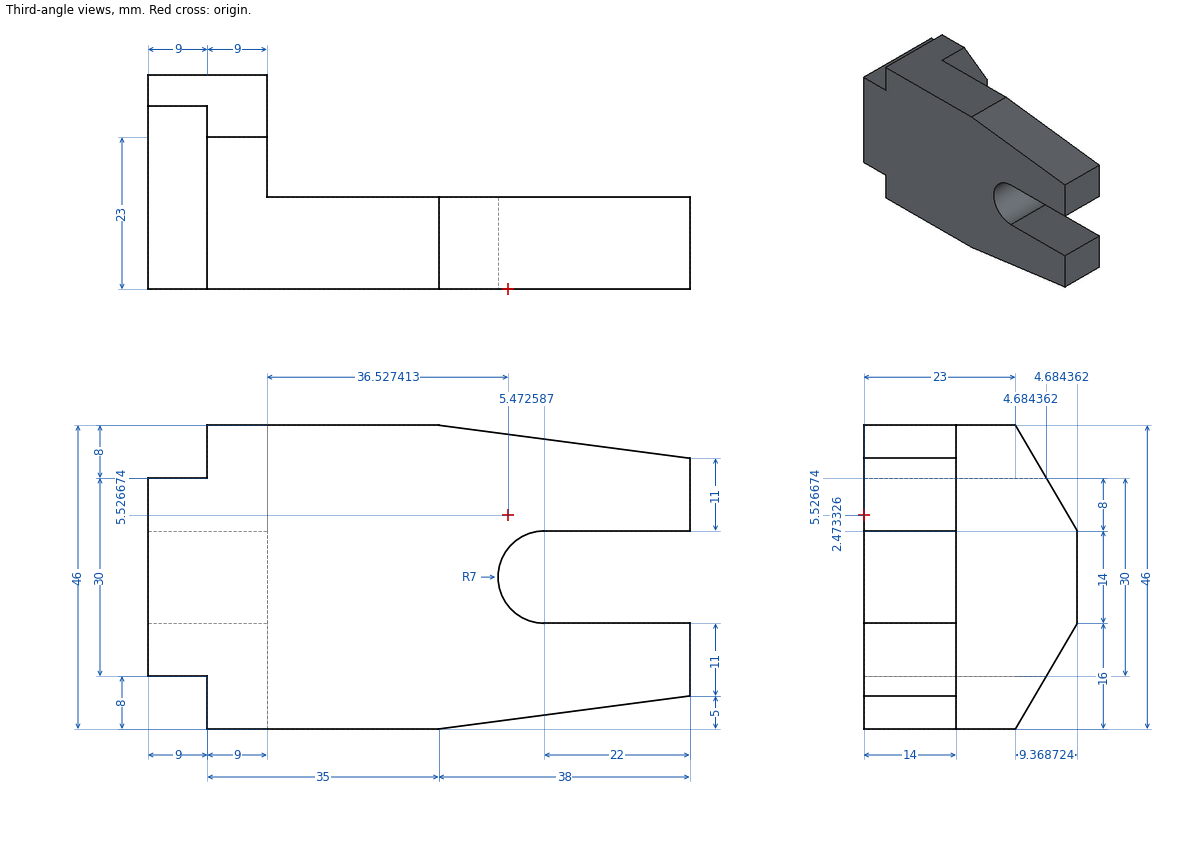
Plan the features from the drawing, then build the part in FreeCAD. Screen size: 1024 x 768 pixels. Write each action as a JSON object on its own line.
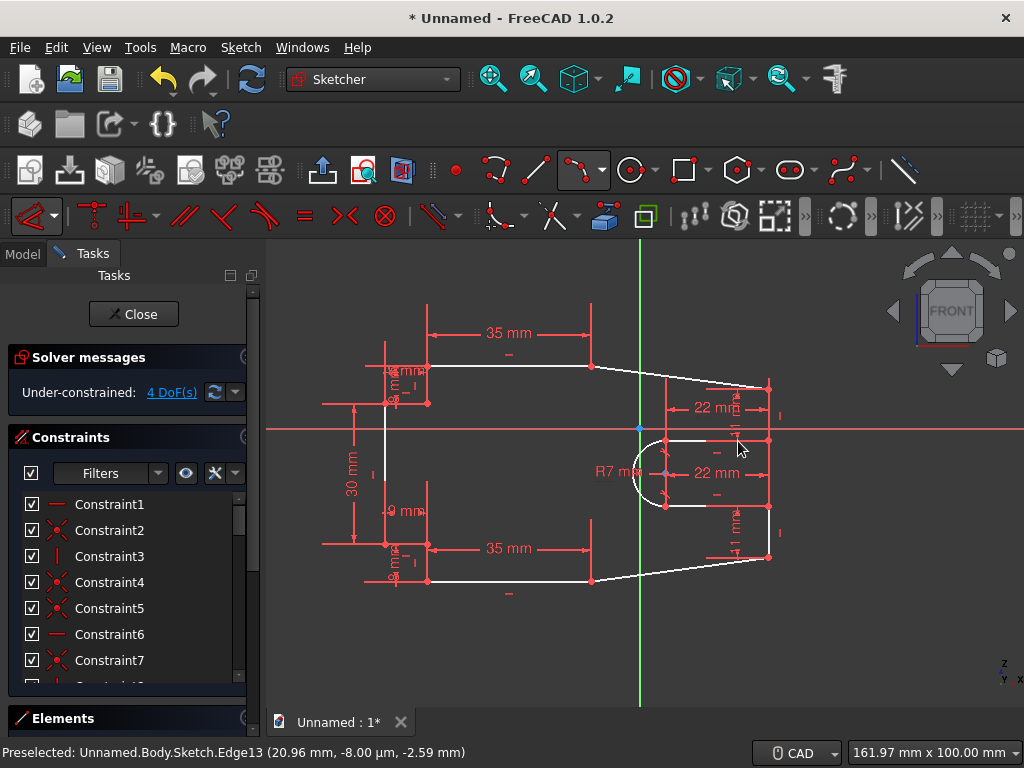
{"action": "scroll", "coordinate": [715, 565], "scroll_direction": "up", "scroll_amount": 3}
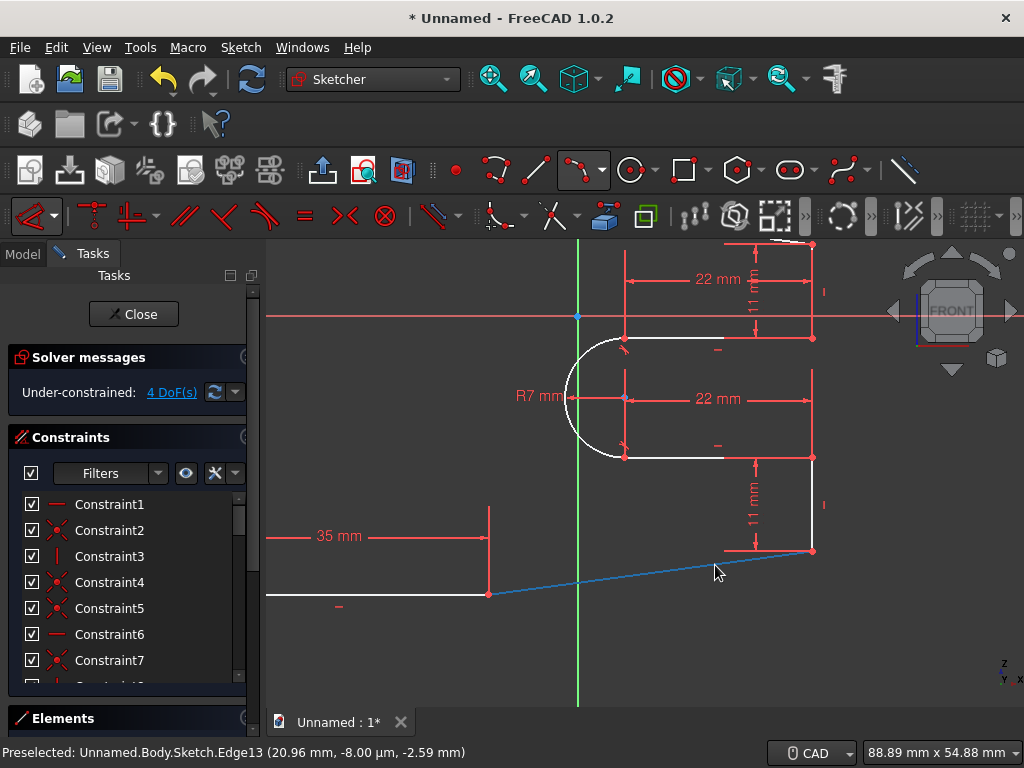
{"action": "left_click", "coordinate": [715, 564]}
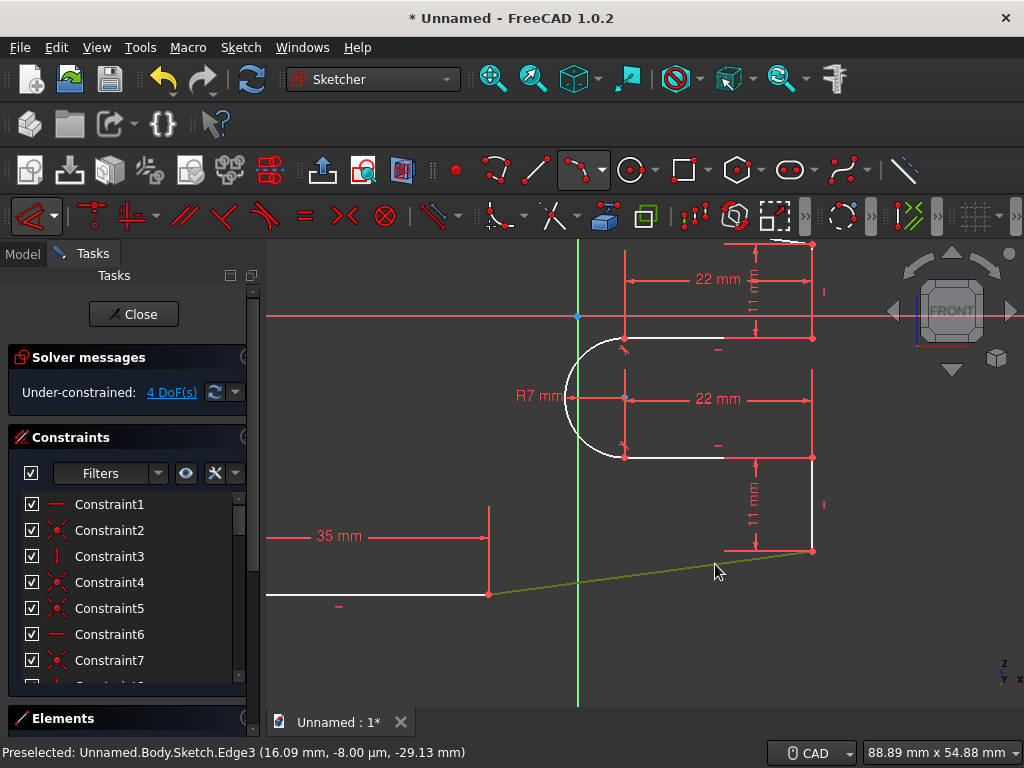
{"action": "left_click", "coordinate": [56, 216]}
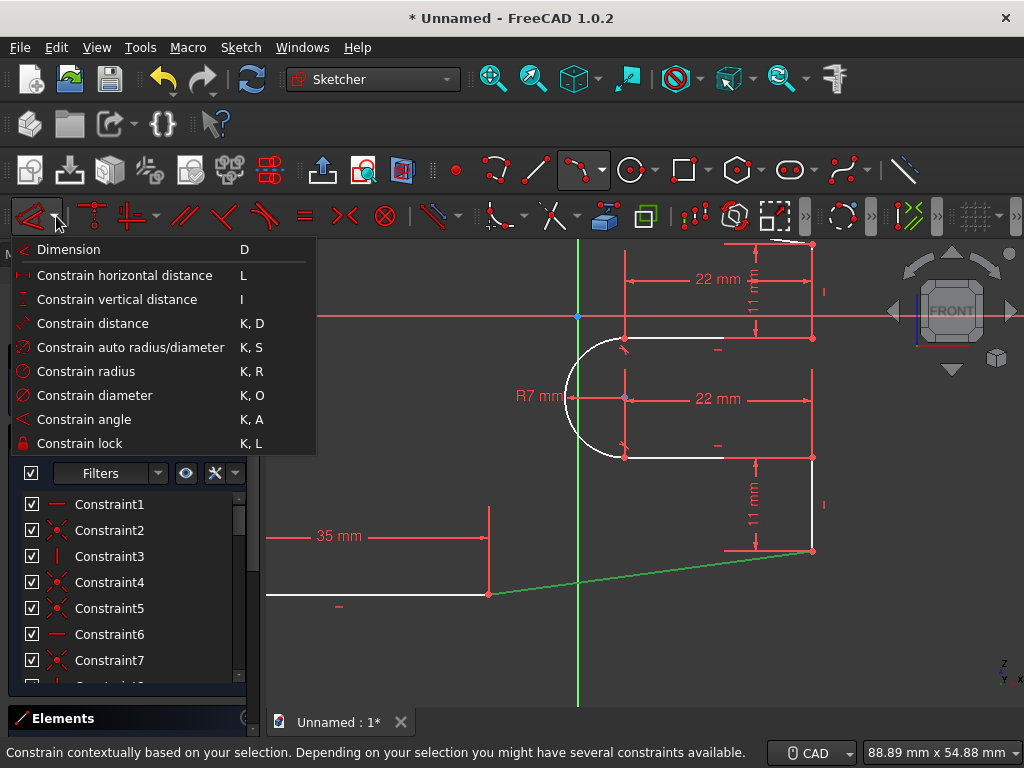
{"action": "left_click", "coordinate": [164, 299]}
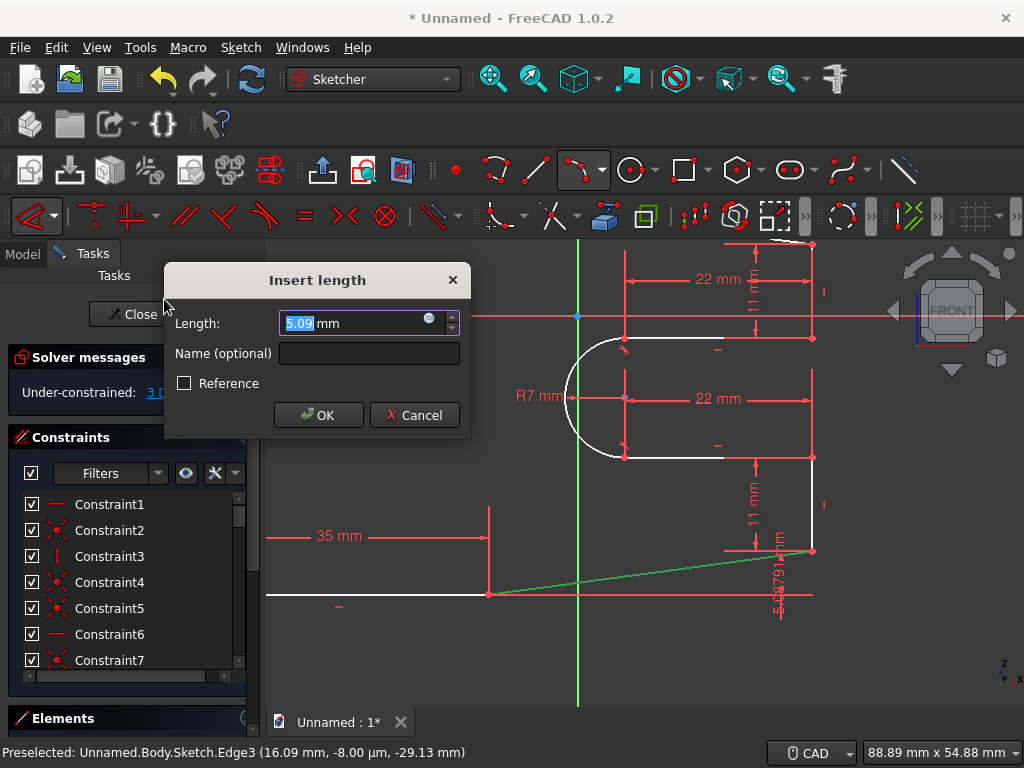
{"action": "type", "text": "5"}
{"action": "key", "text": "Return"}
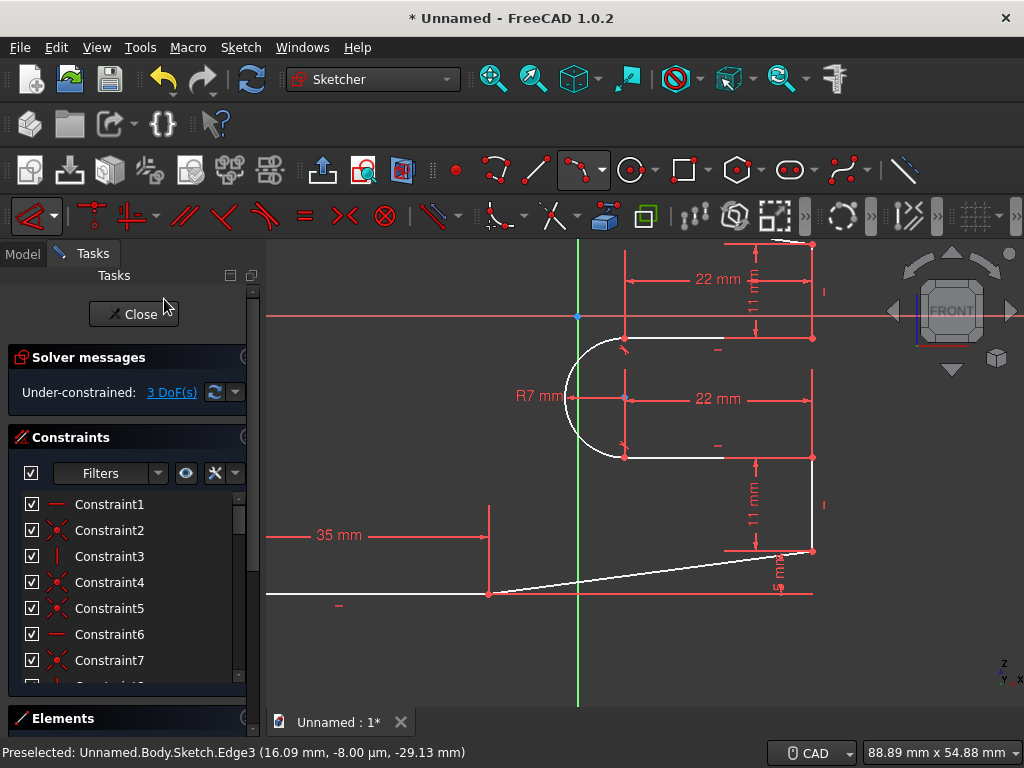
{"action": "left_click", "coordinate": [715, 564]}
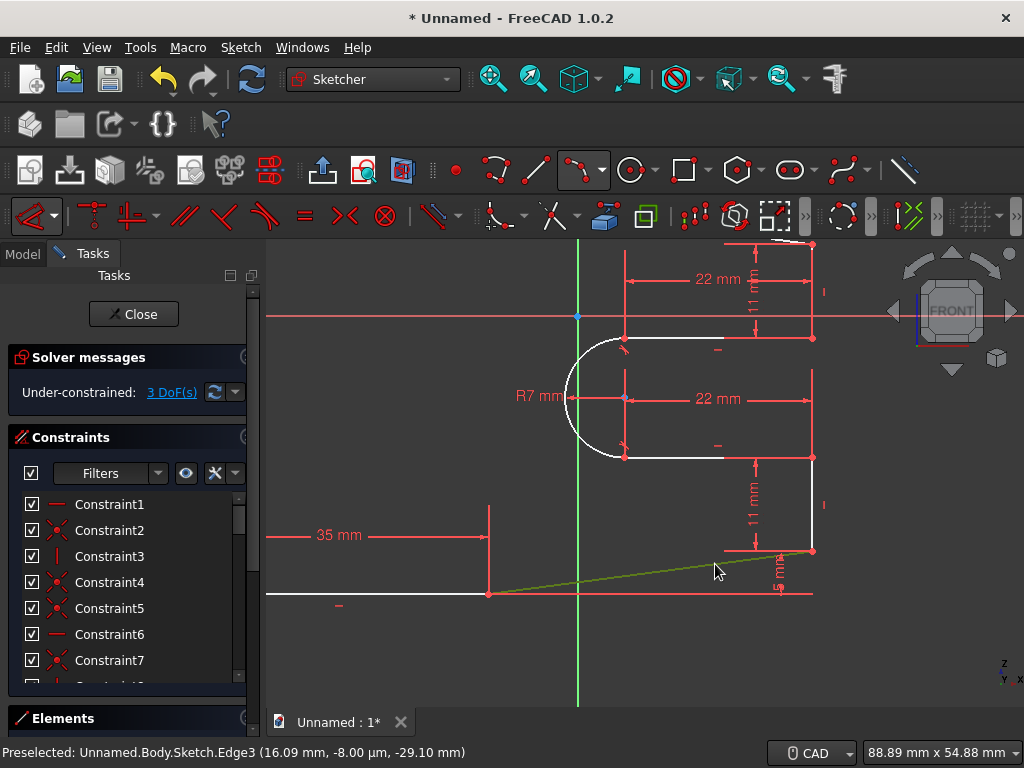
{"action": "key", "text": "l"}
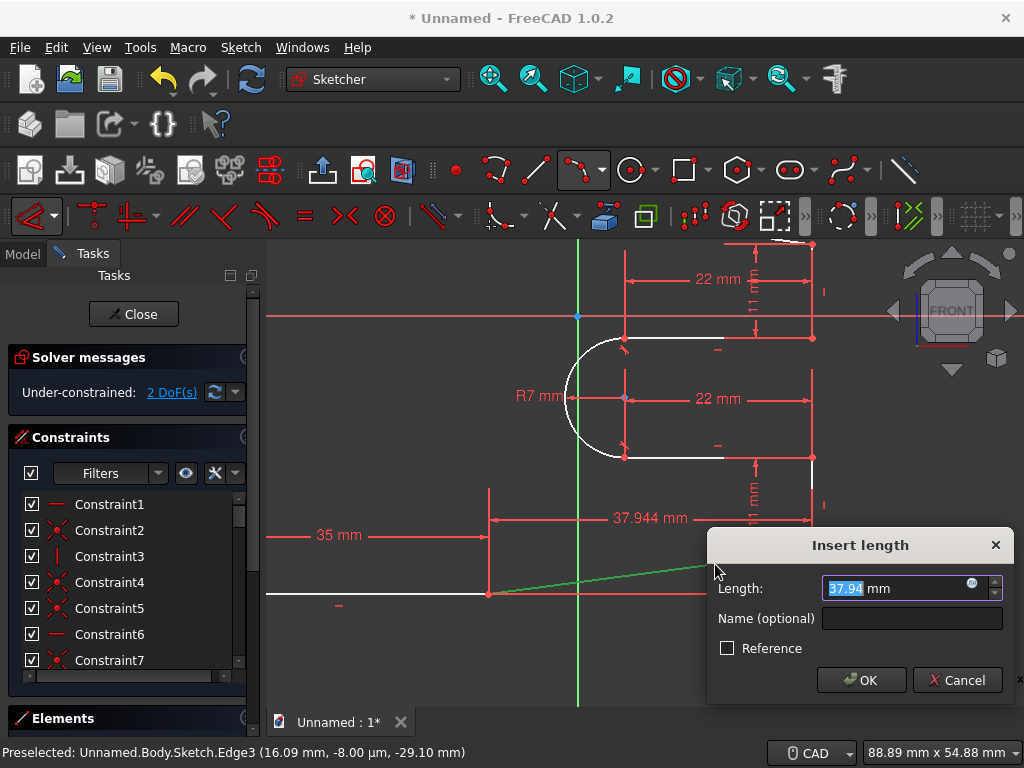
{"action": "type", "text": "38"}
{"action": "key", "text": "Return"}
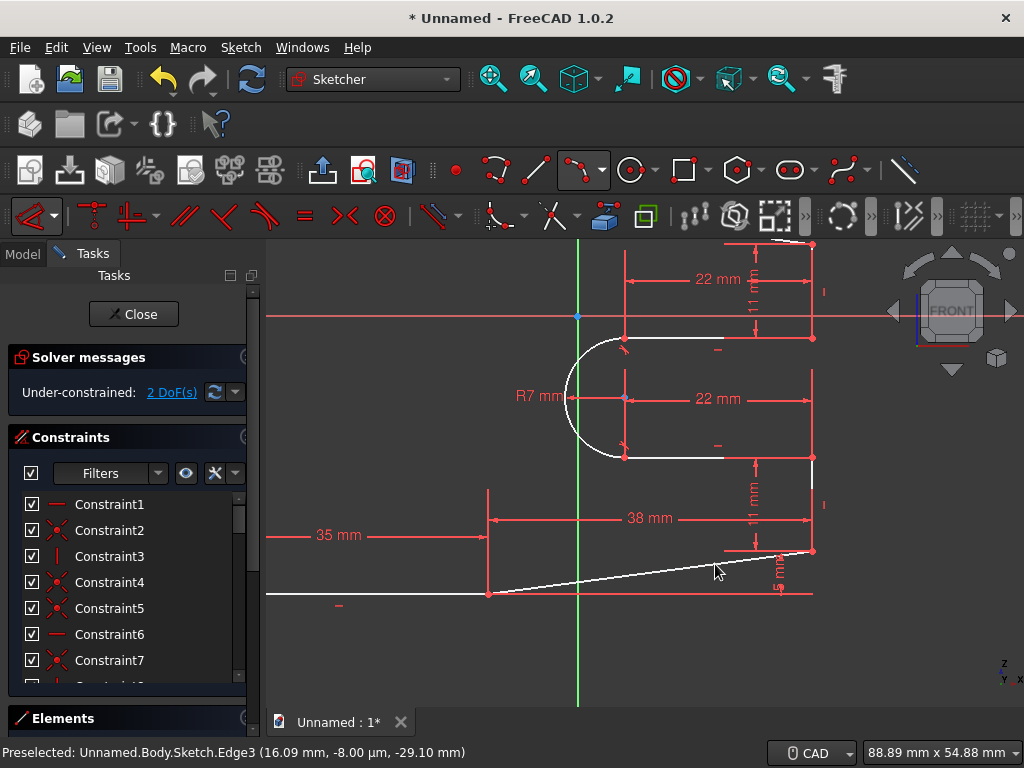
{"action": "left_click", "coordinate": [625, 458]}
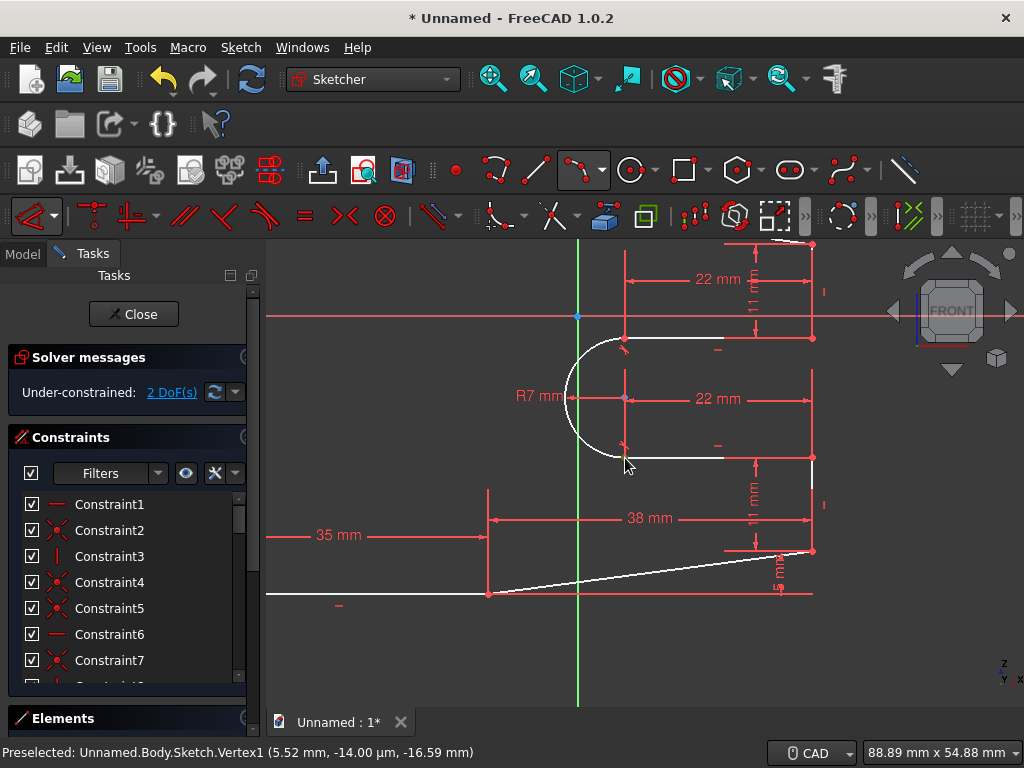
{"action": "key", "text": "l"}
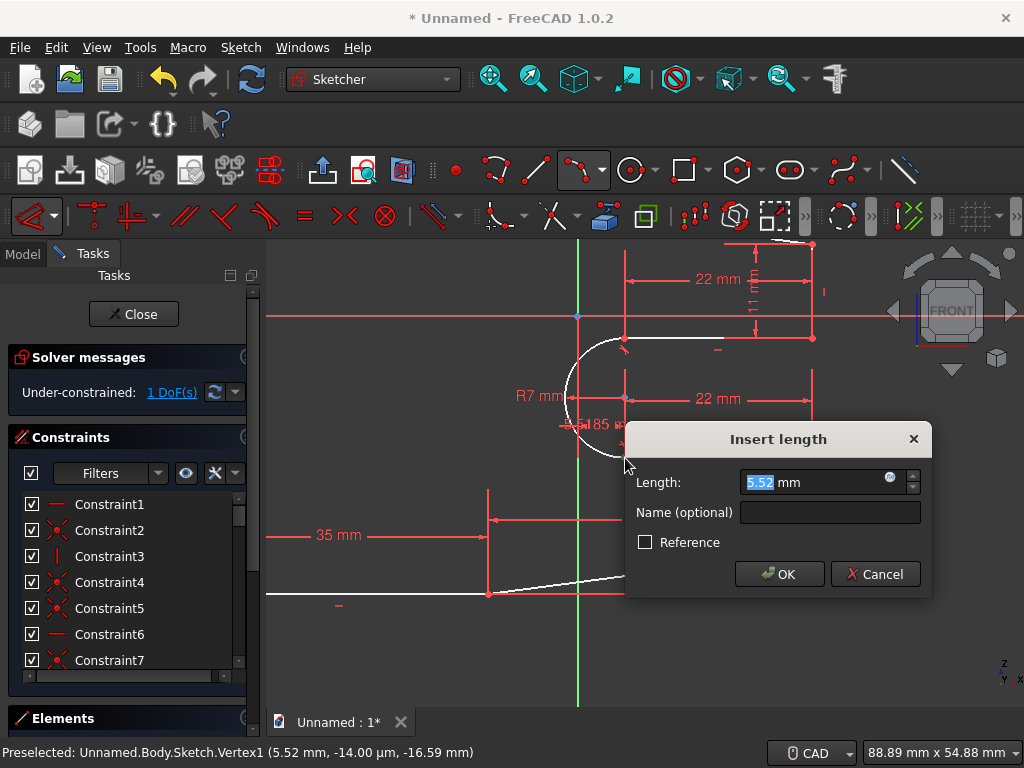
{"action": "type", "text": "5.472587"}
{"action": "key", "text": "Return"}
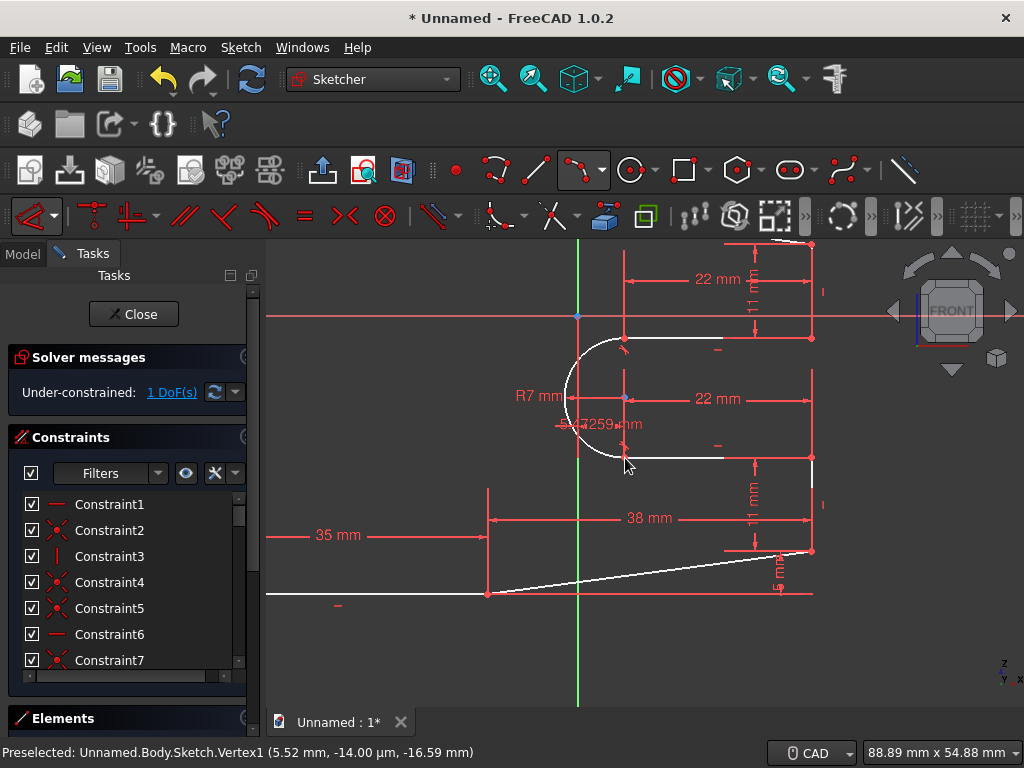
{"action": "scroll", "coordinate": [715, 566], "scroll_direction": "down", "scroll_amount": 3}